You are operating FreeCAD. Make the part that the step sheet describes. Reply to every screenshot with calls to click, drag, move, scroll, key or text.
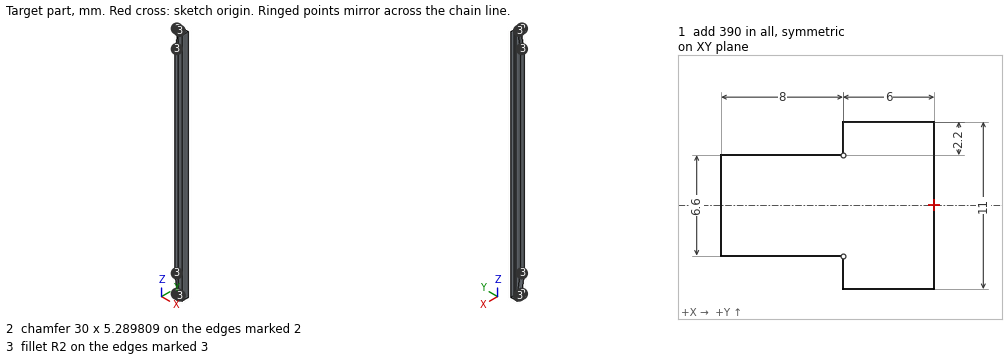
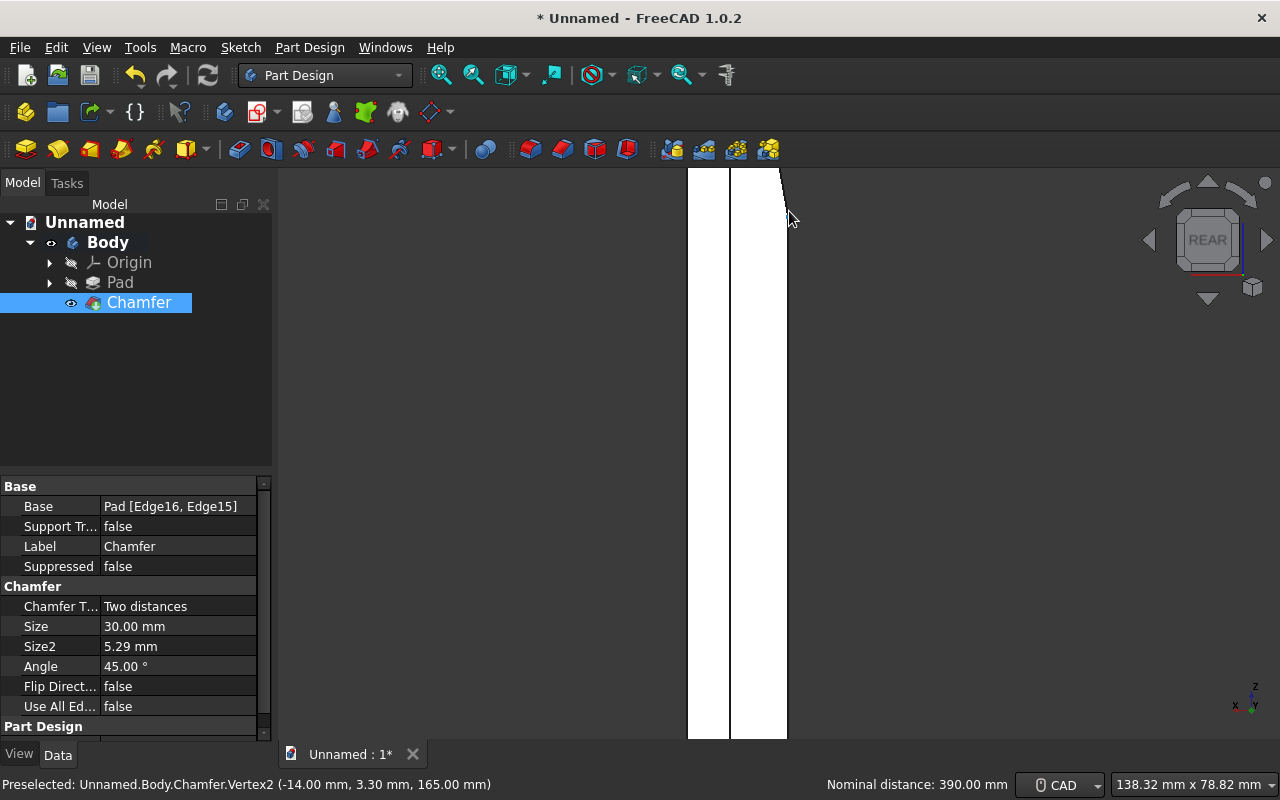
click(442, 76)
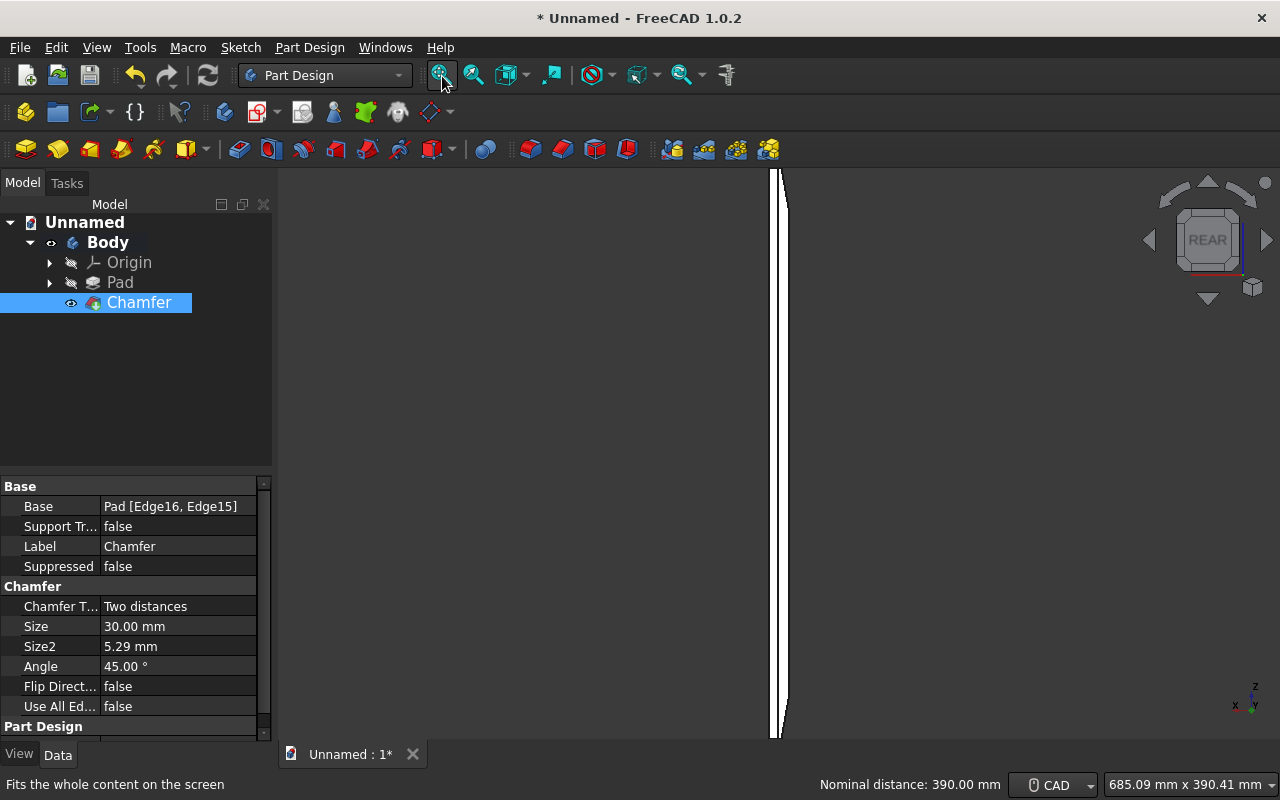
key(6)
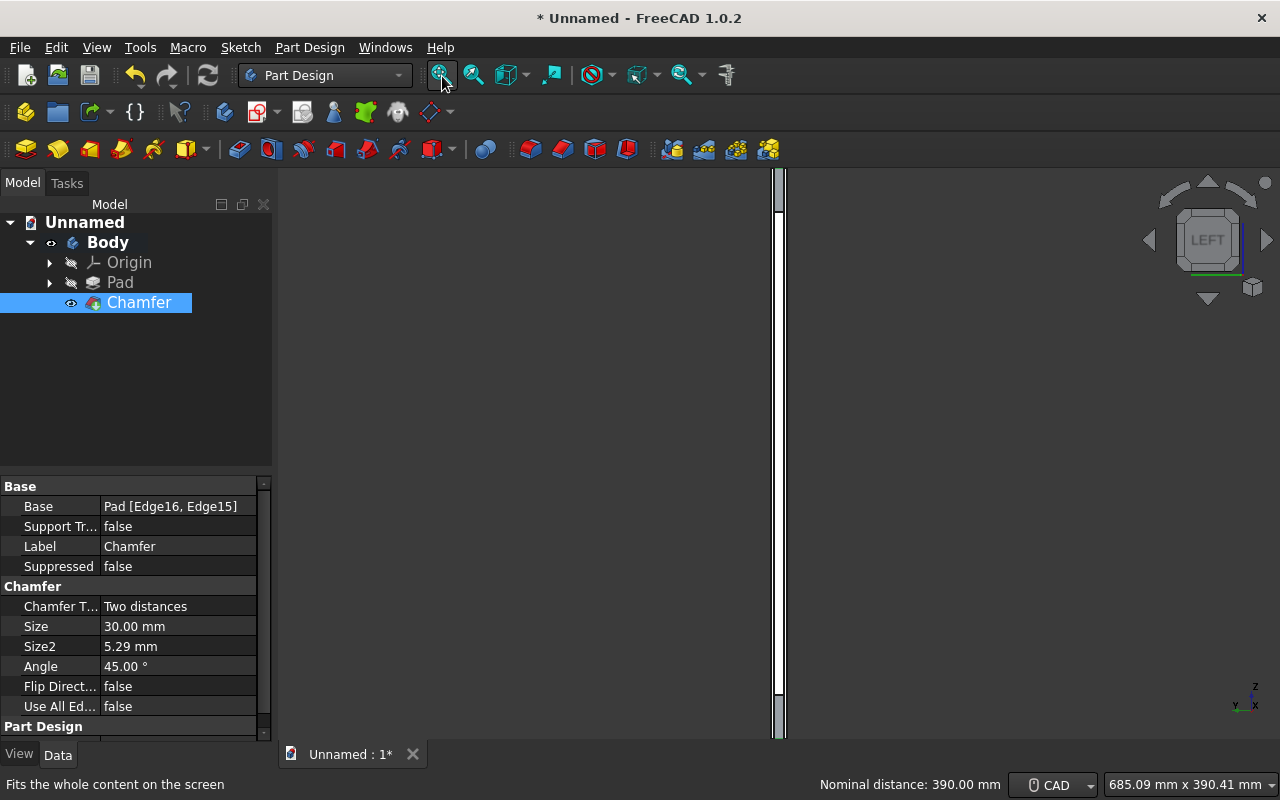
click(442, 76)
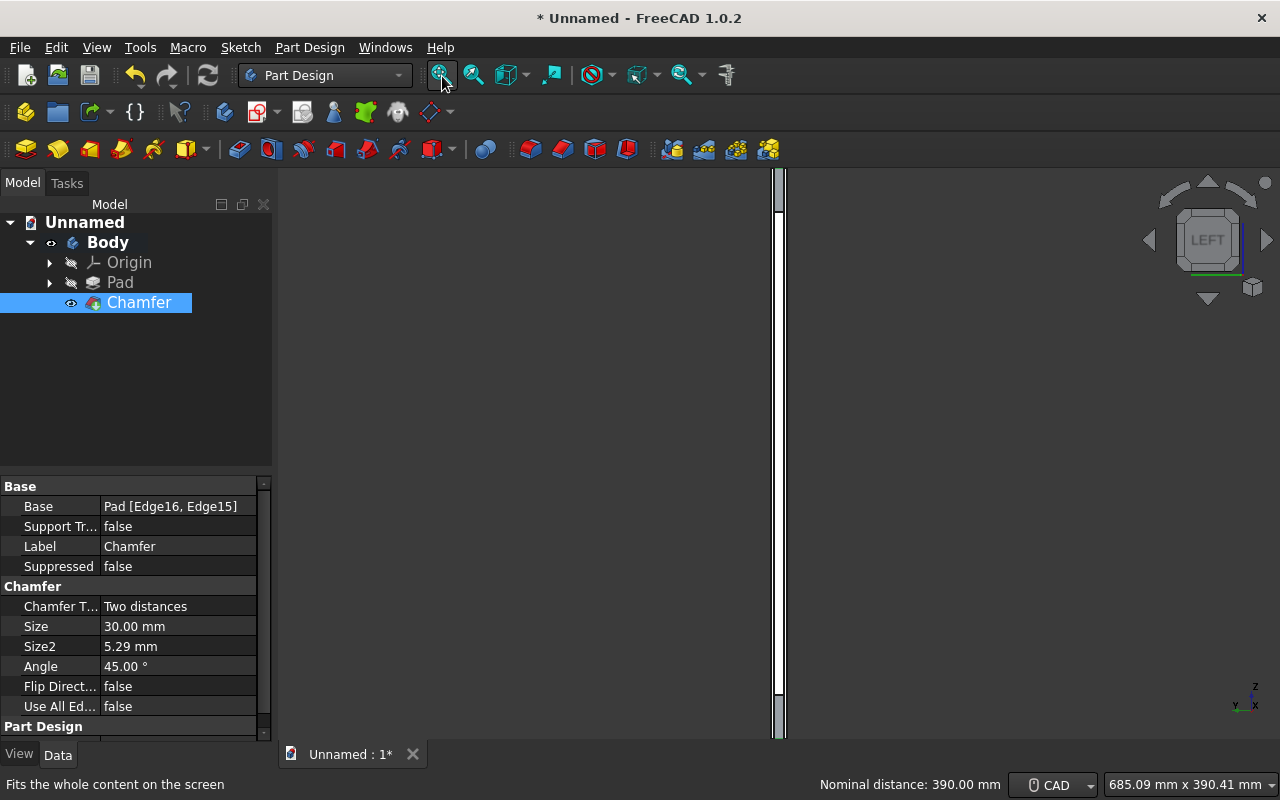
scroll(779, 211, up, 8)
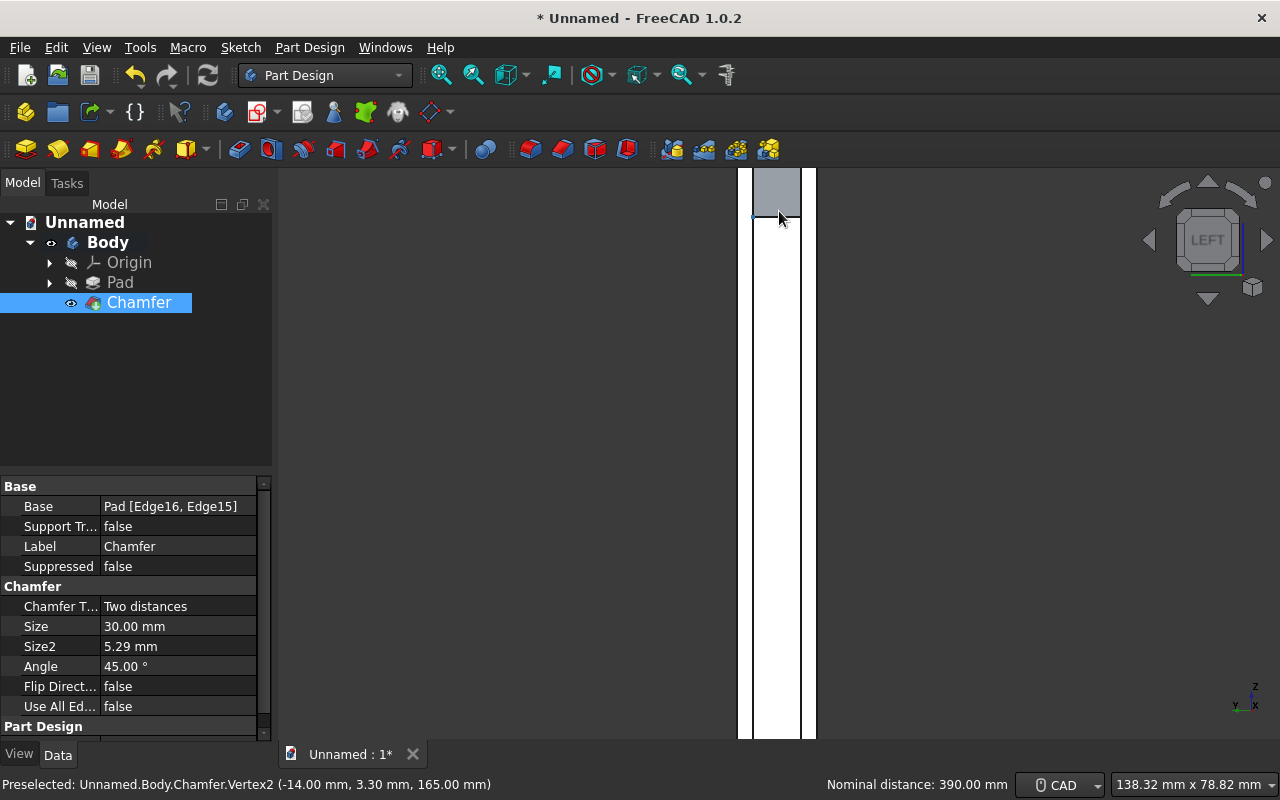
click(777, 216, ctrl)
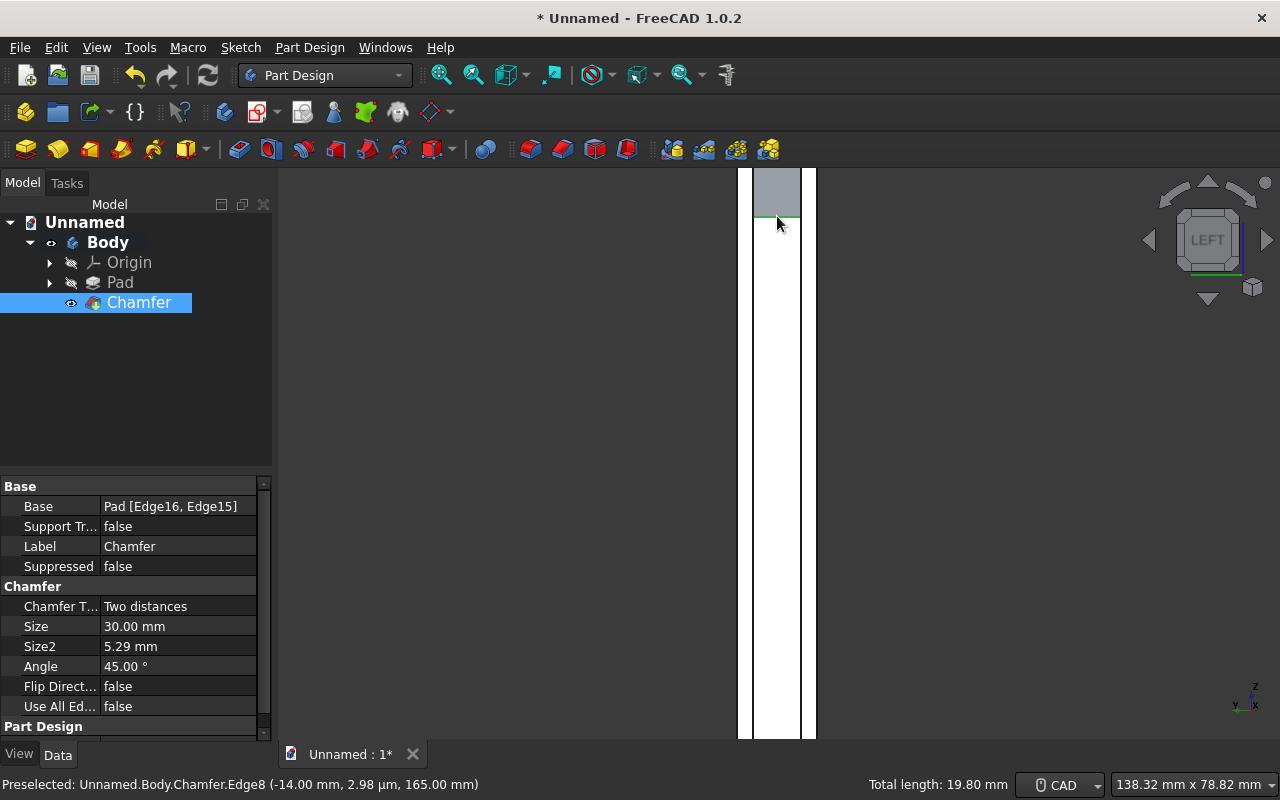
click(442, 76)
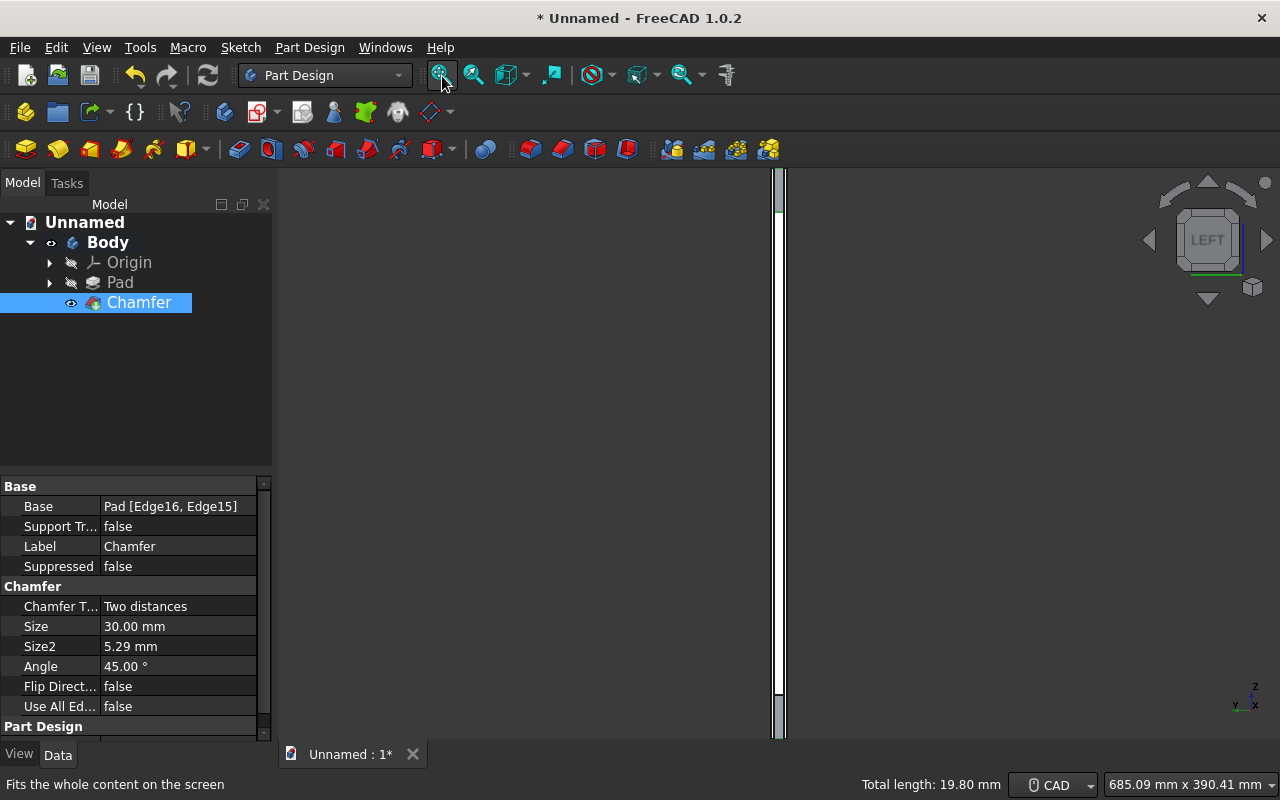
key(v)
key(3)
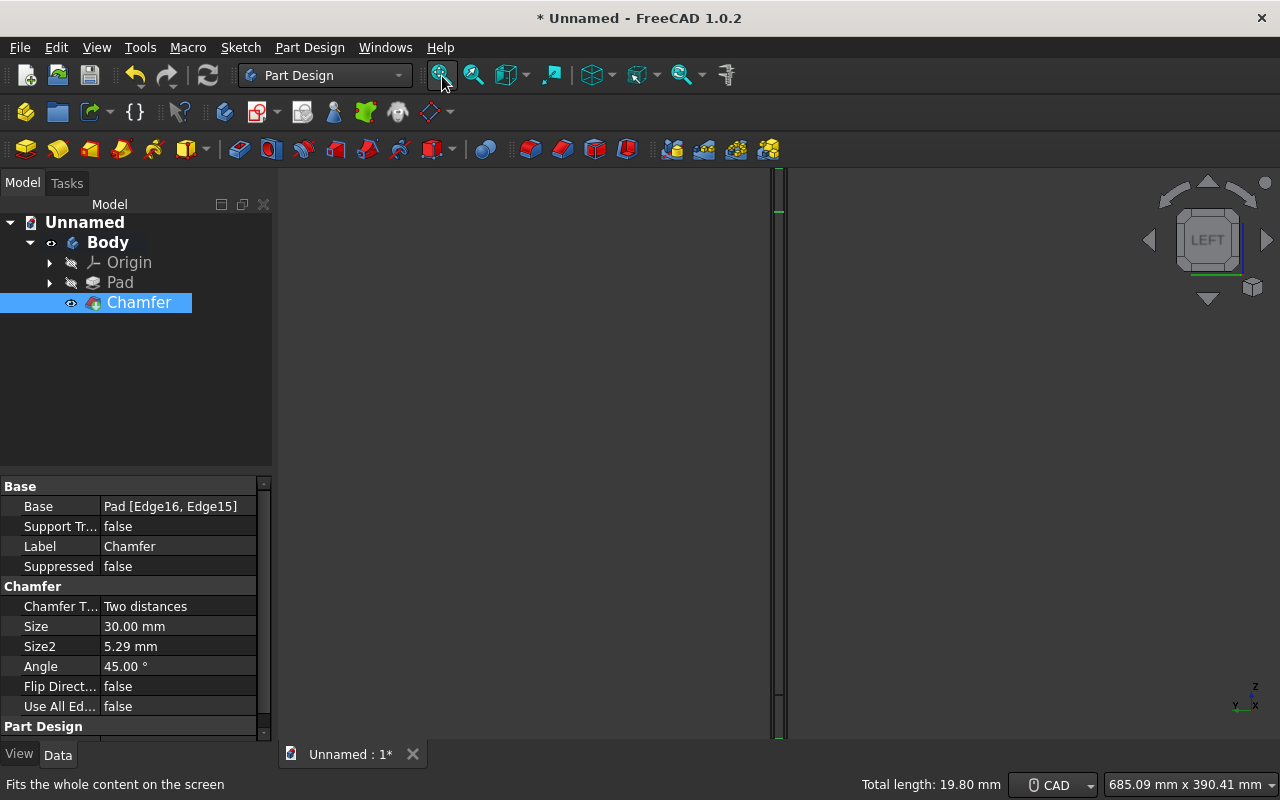
key(0)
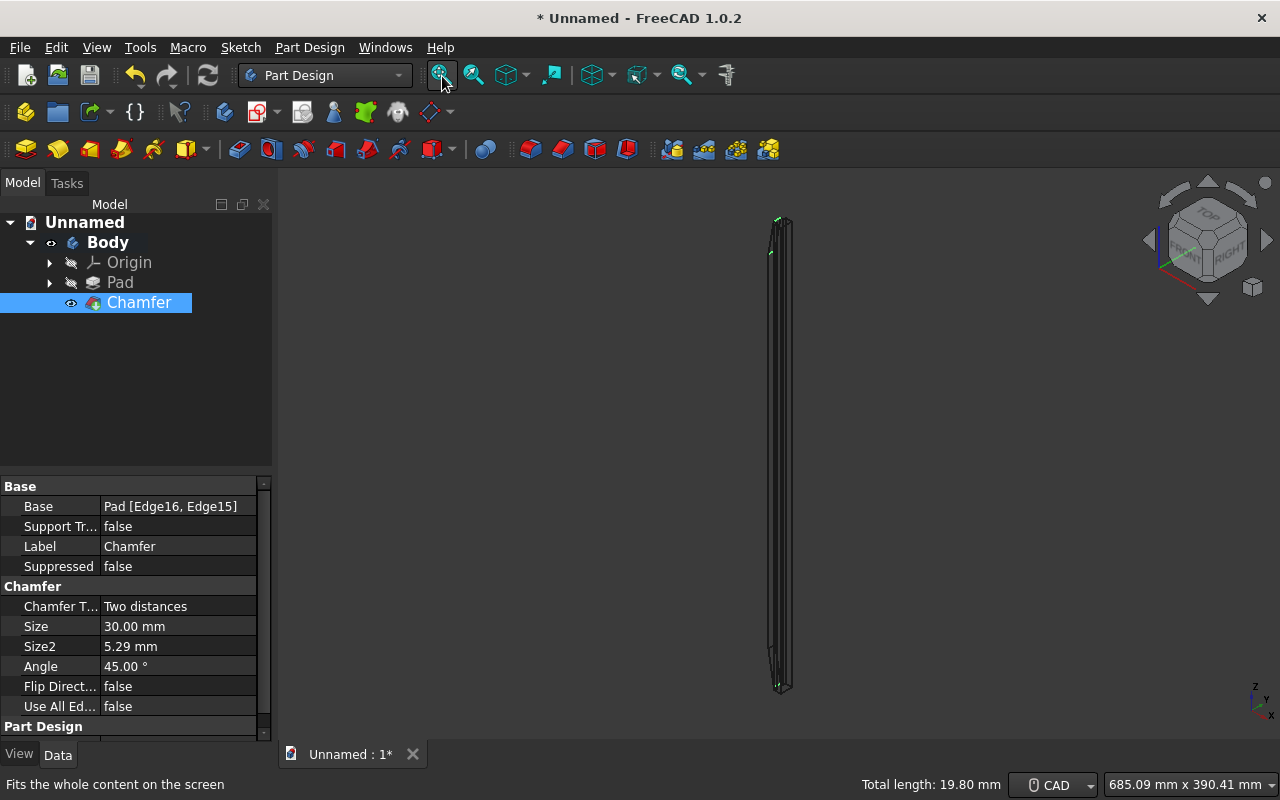
scroll(772, 645, up, 8)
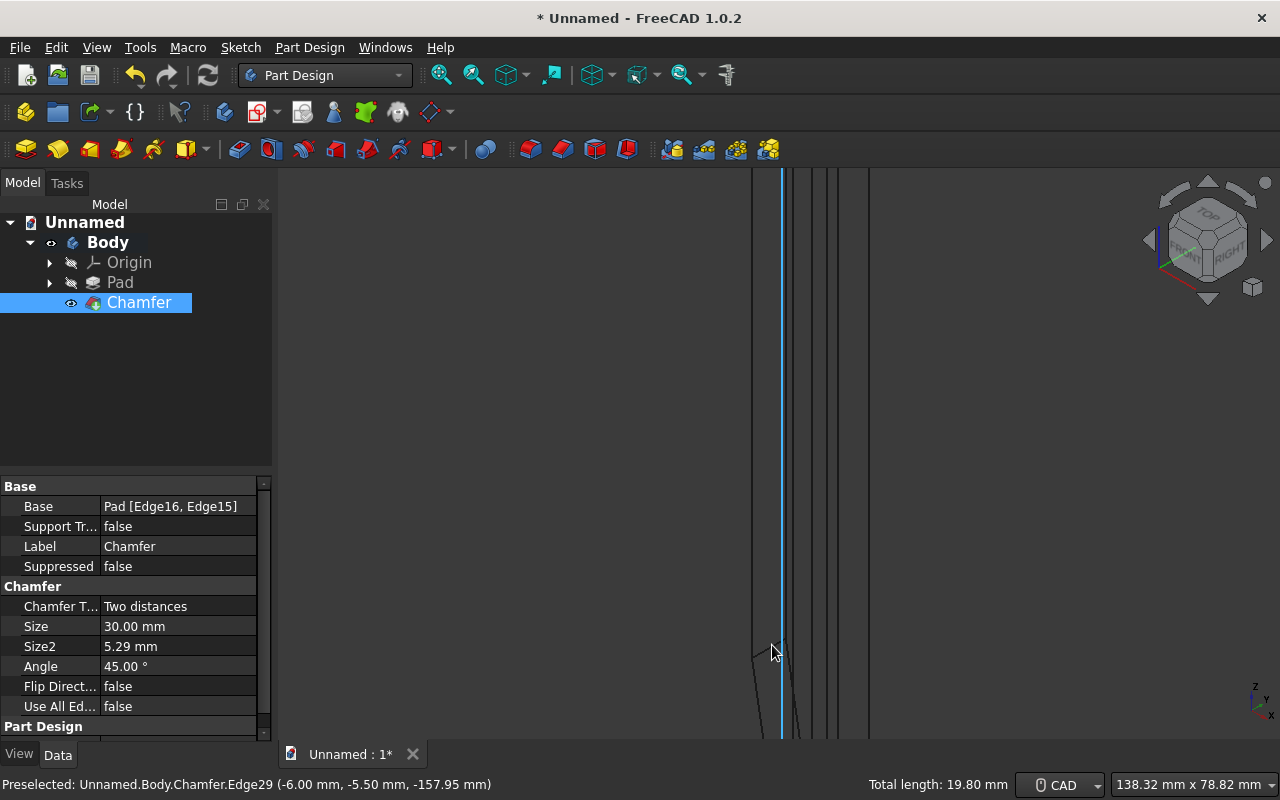
click(769, 647, ctrl)